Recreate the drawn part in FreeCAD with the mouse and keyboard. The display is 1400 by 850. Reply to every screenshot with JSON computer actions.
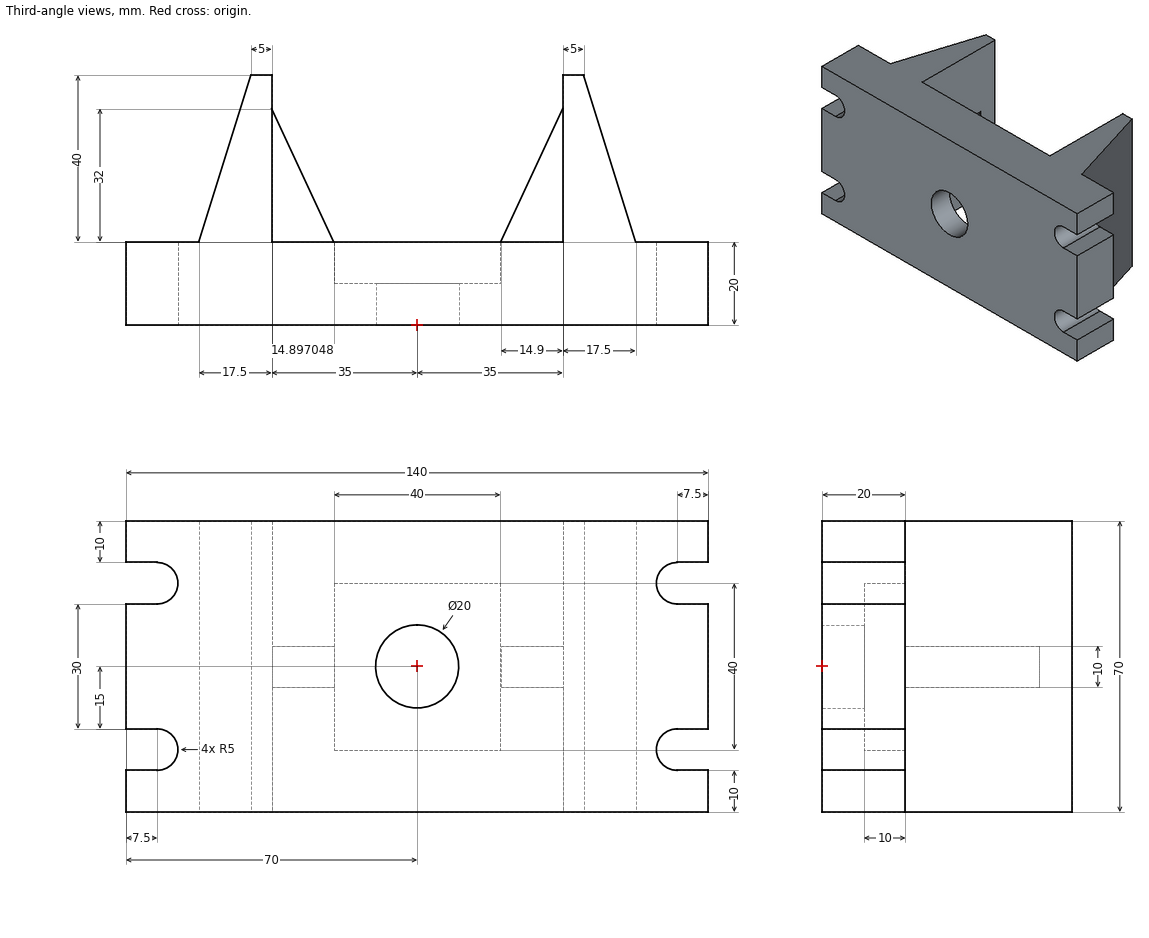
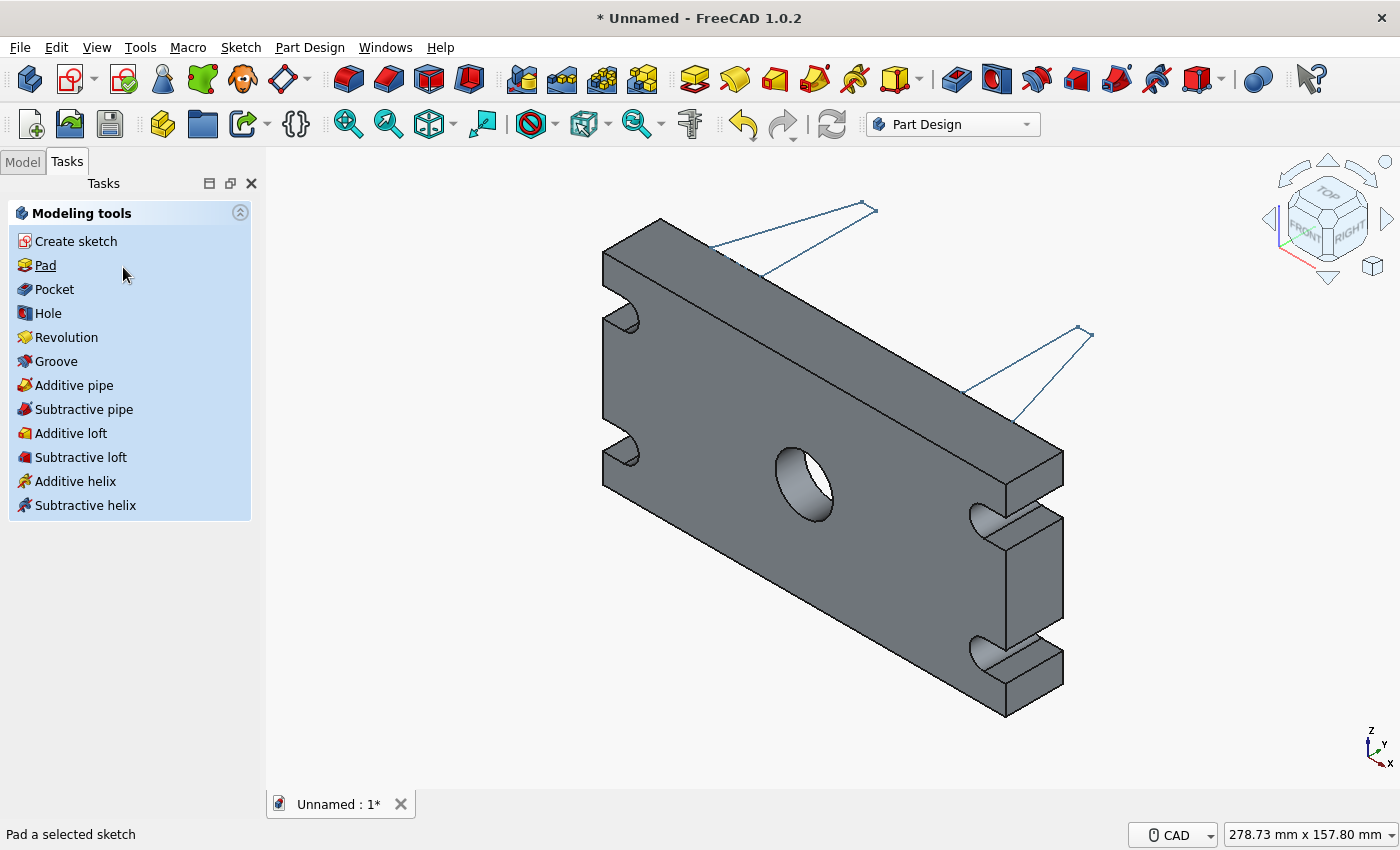
{"action": "left_click", "coordinate": [696, 80]}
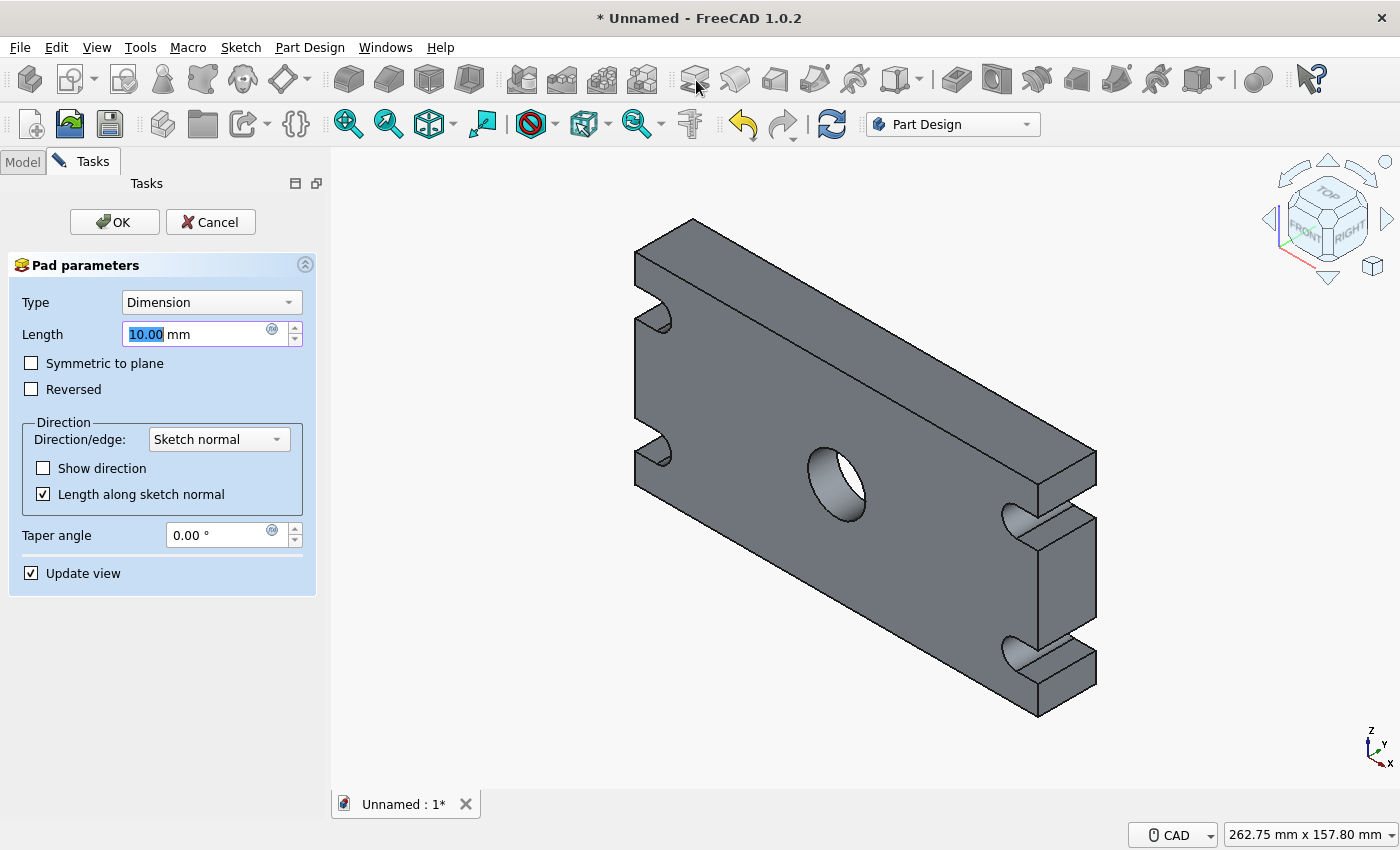
{"action": "type", "text": "70"}
{"action": "key", "text": "Tab"}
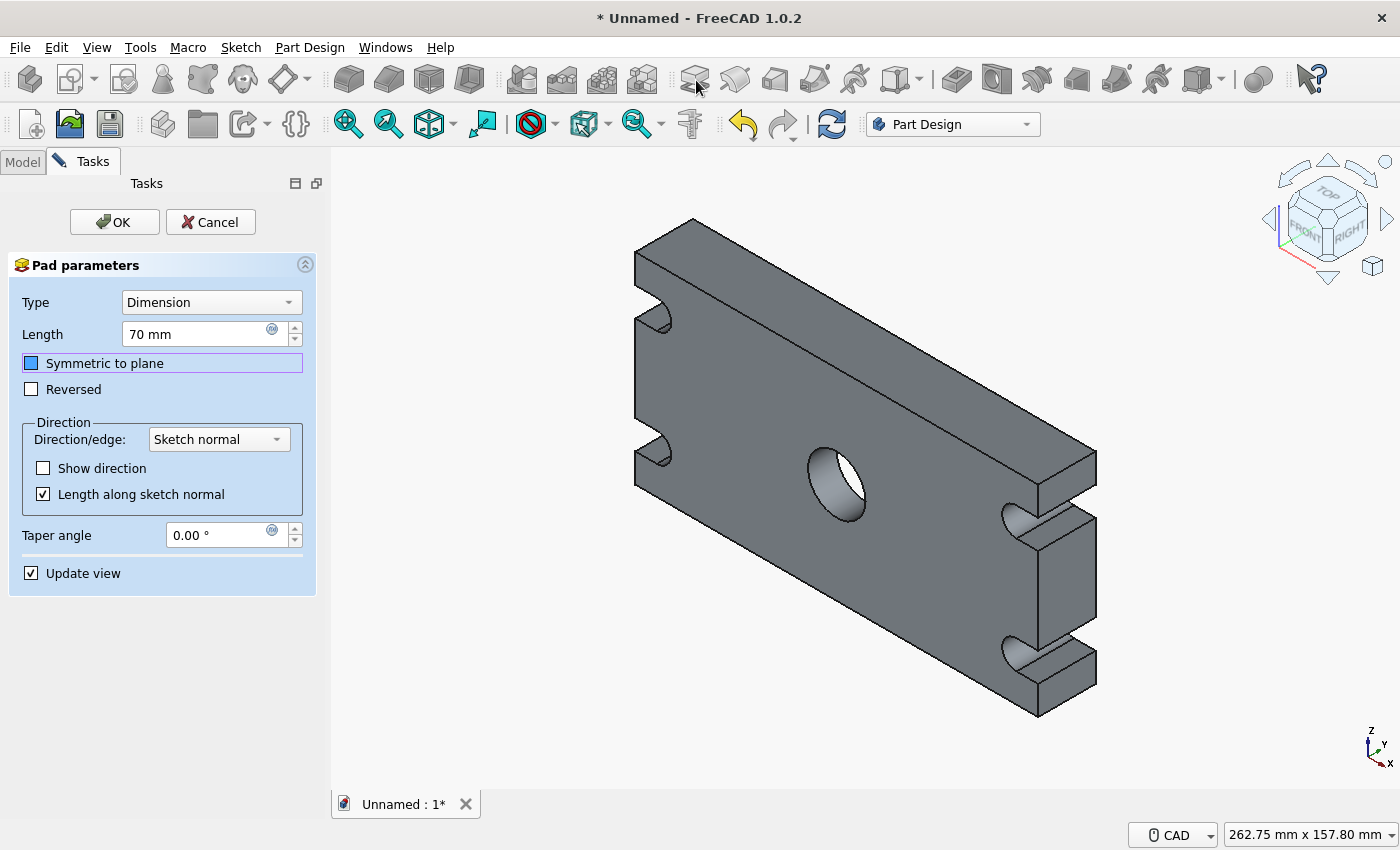
{"action": "left_click", "coordinate": [30, 389]}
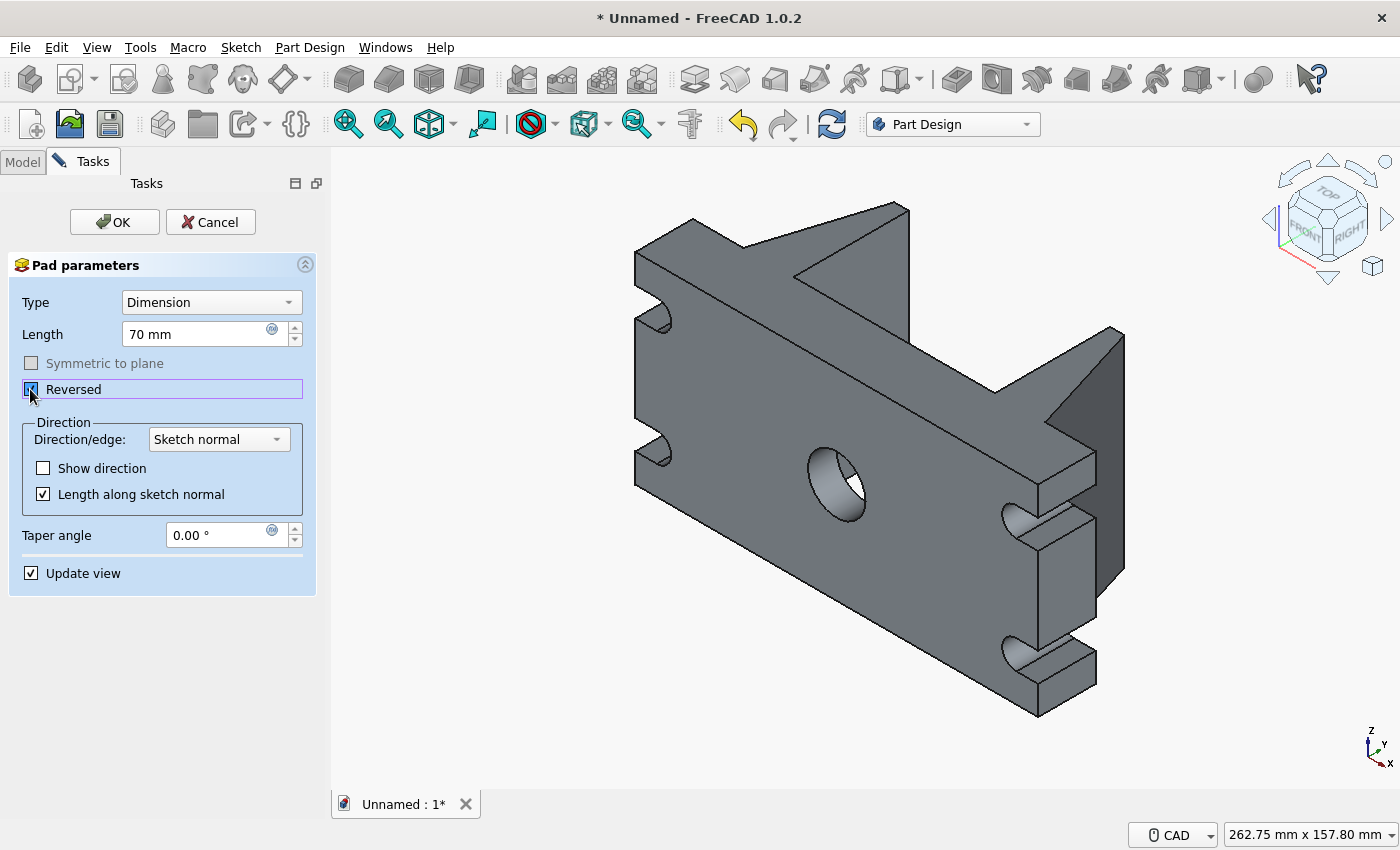
{"action": "left_click", "coordinate": [115, 222]}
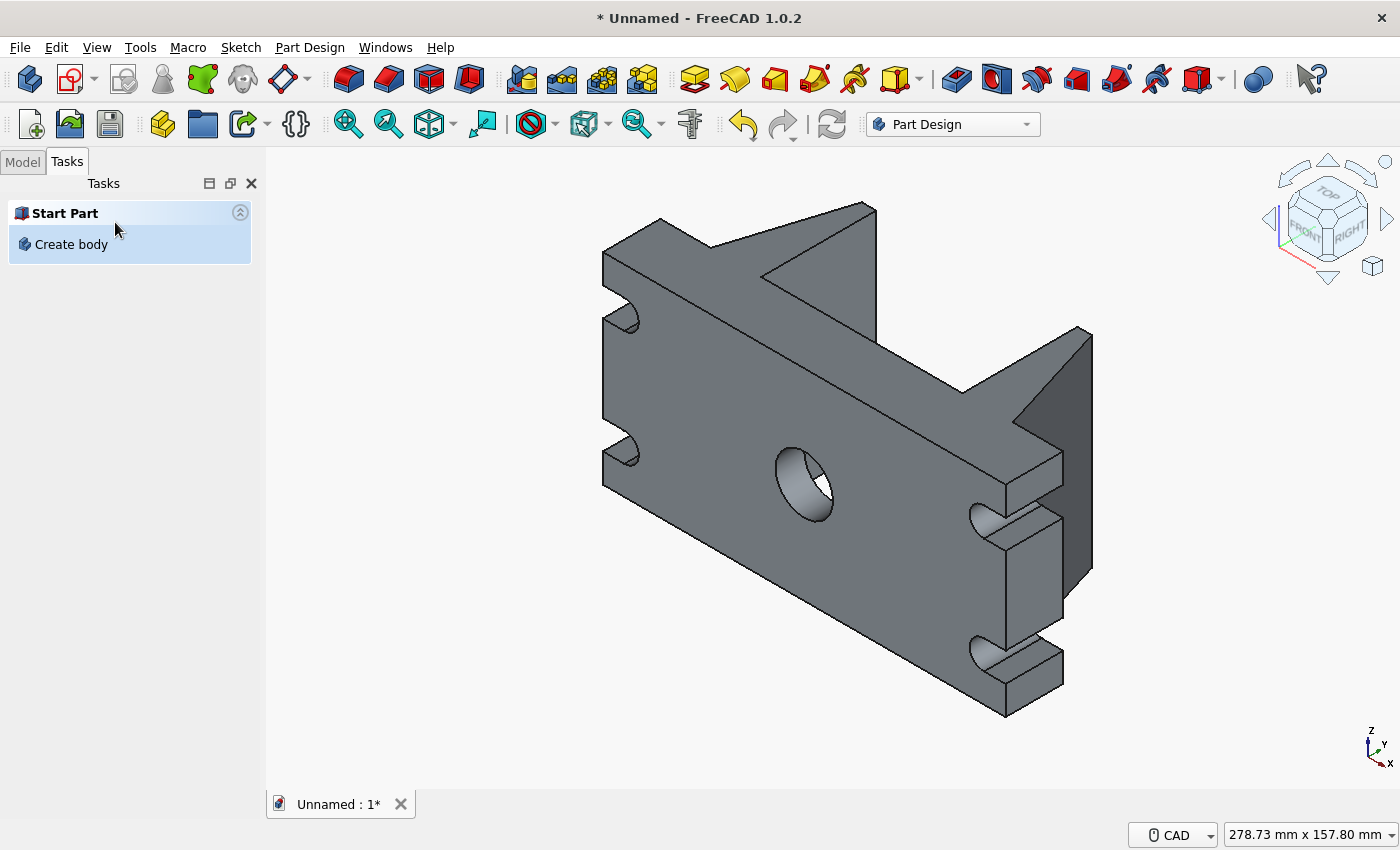
{"action": "left_click", "coordinate": [70, 80]}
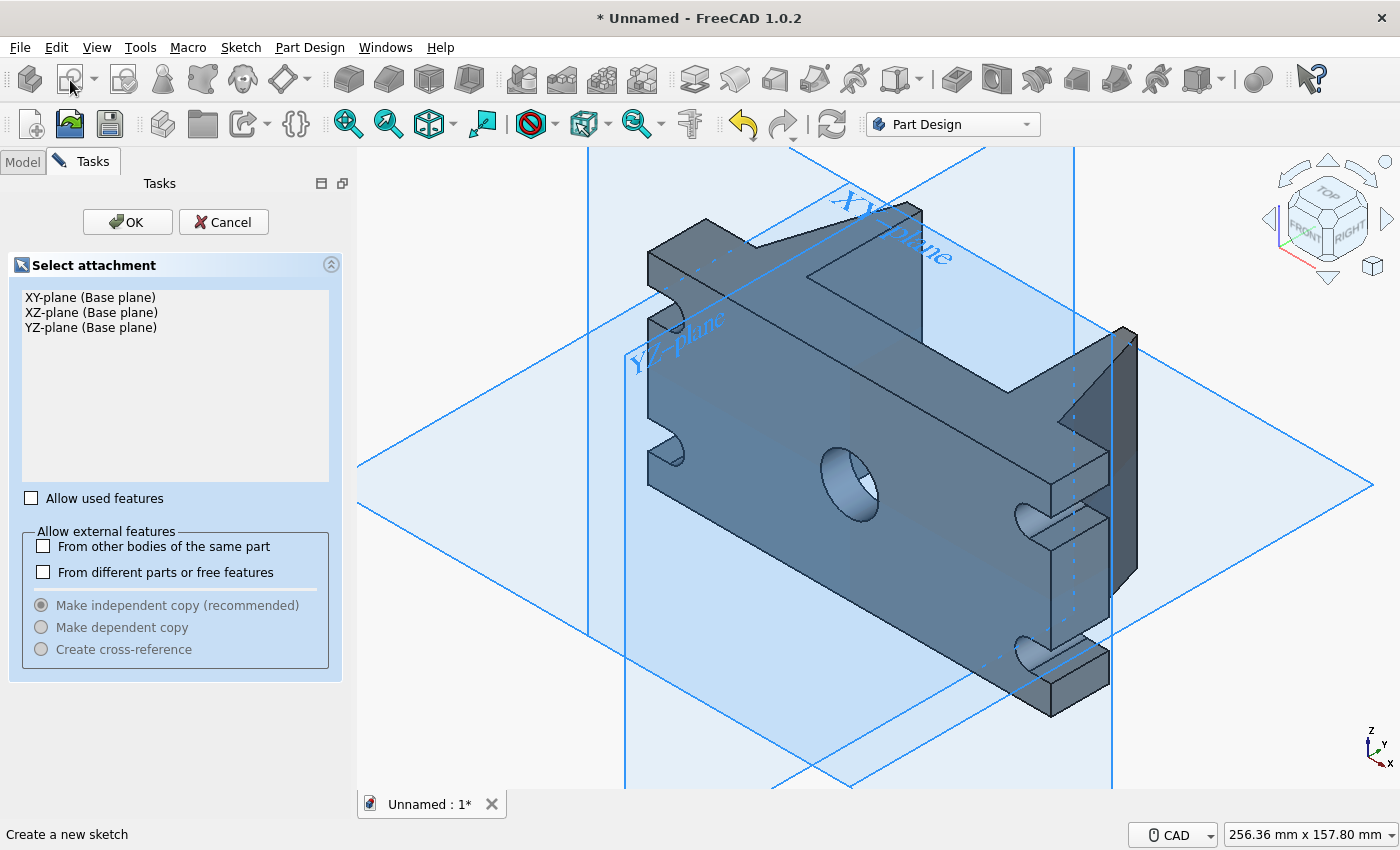
{"action": "left_click", "coordinate": [82, 298]}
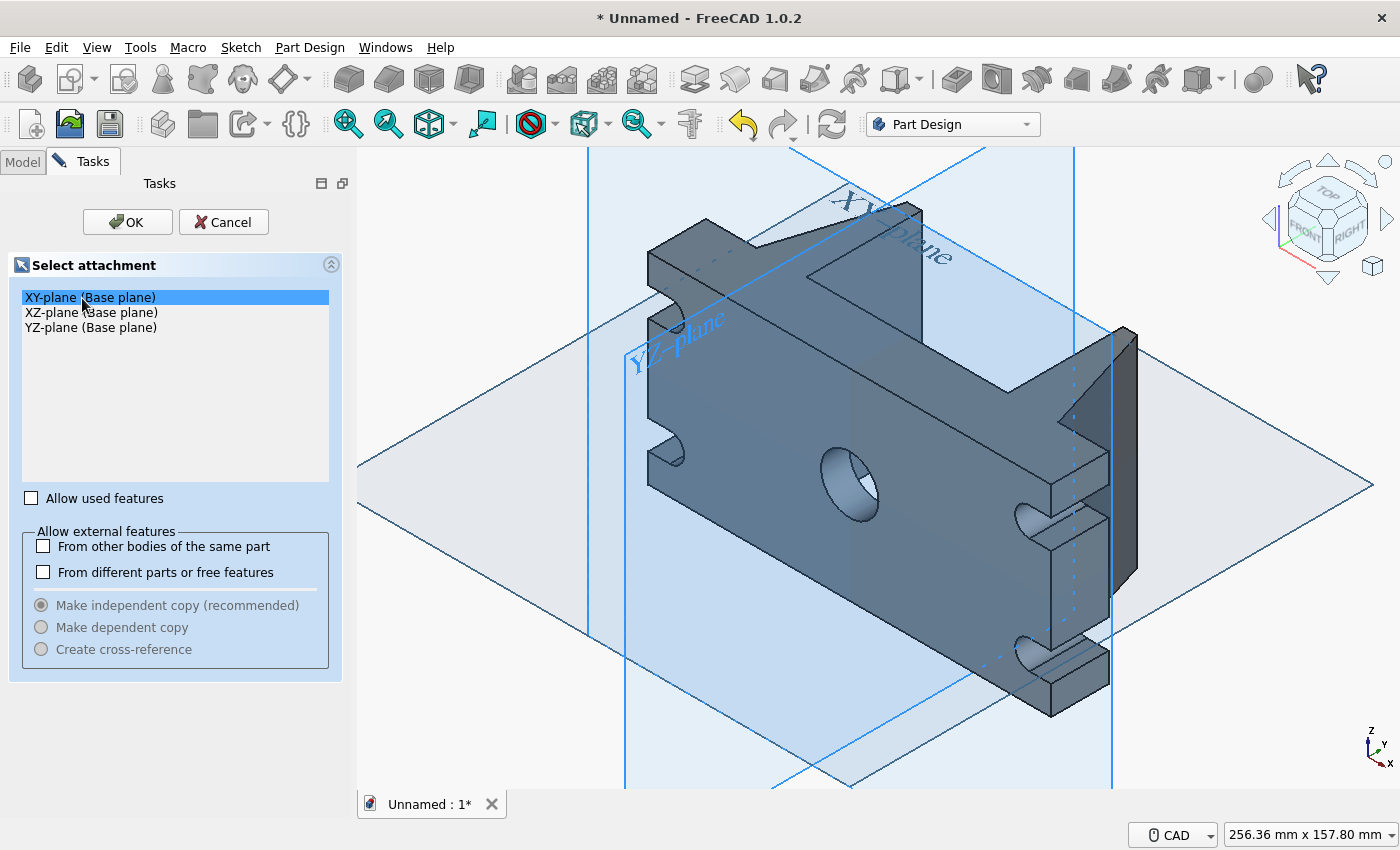
{"action": "left_click", "coordinate": [128, 222]}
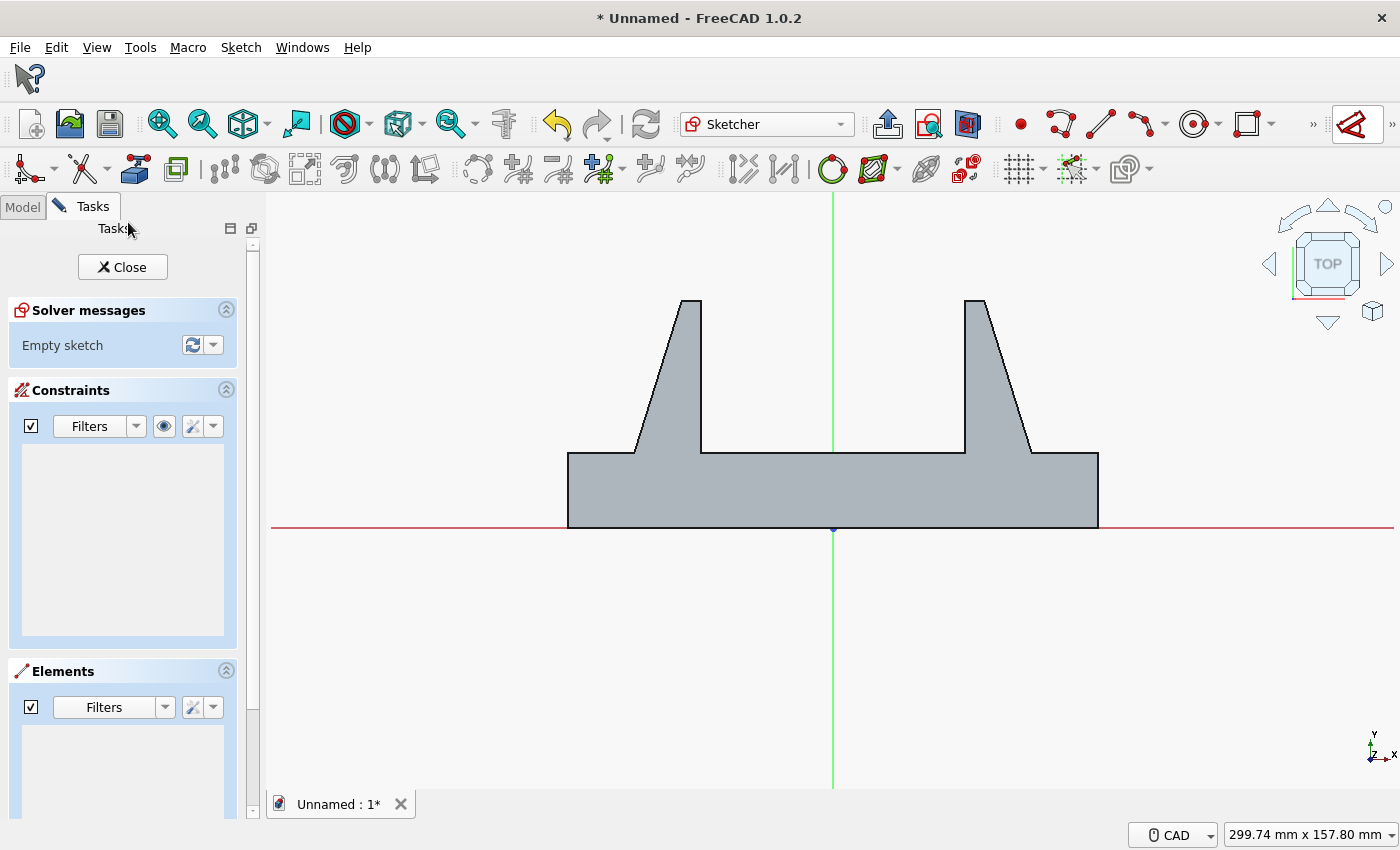
{"action": "left_click", "coordinate": [968, 124]}